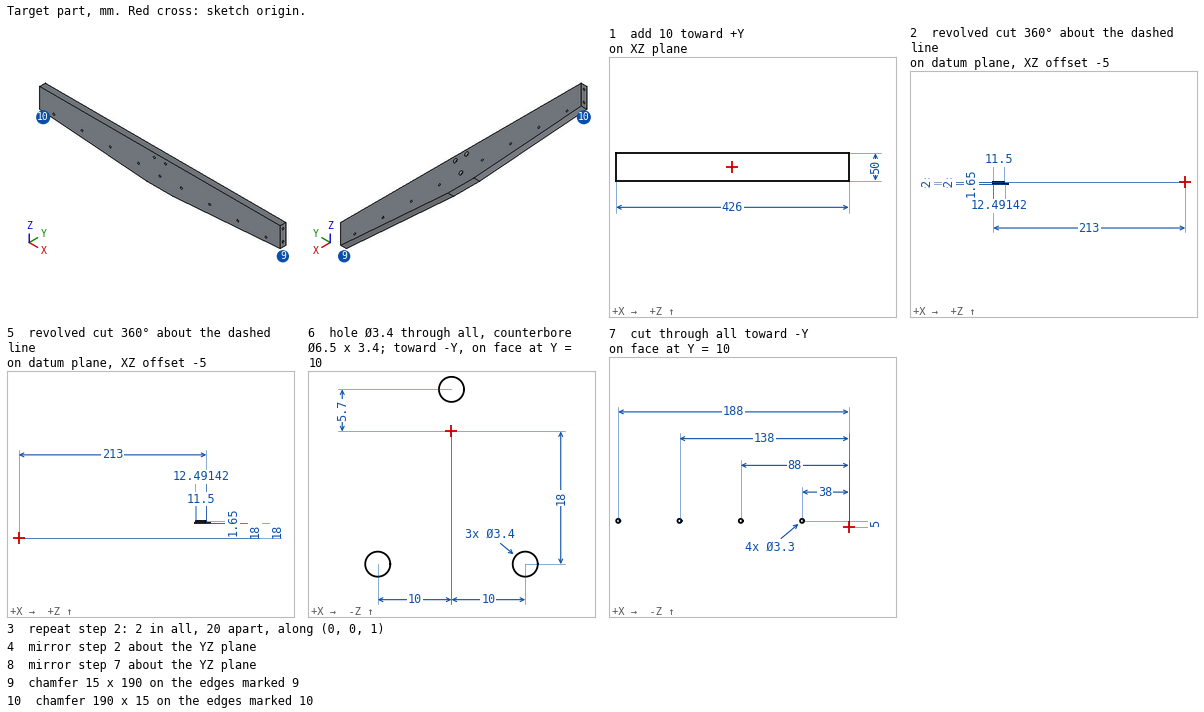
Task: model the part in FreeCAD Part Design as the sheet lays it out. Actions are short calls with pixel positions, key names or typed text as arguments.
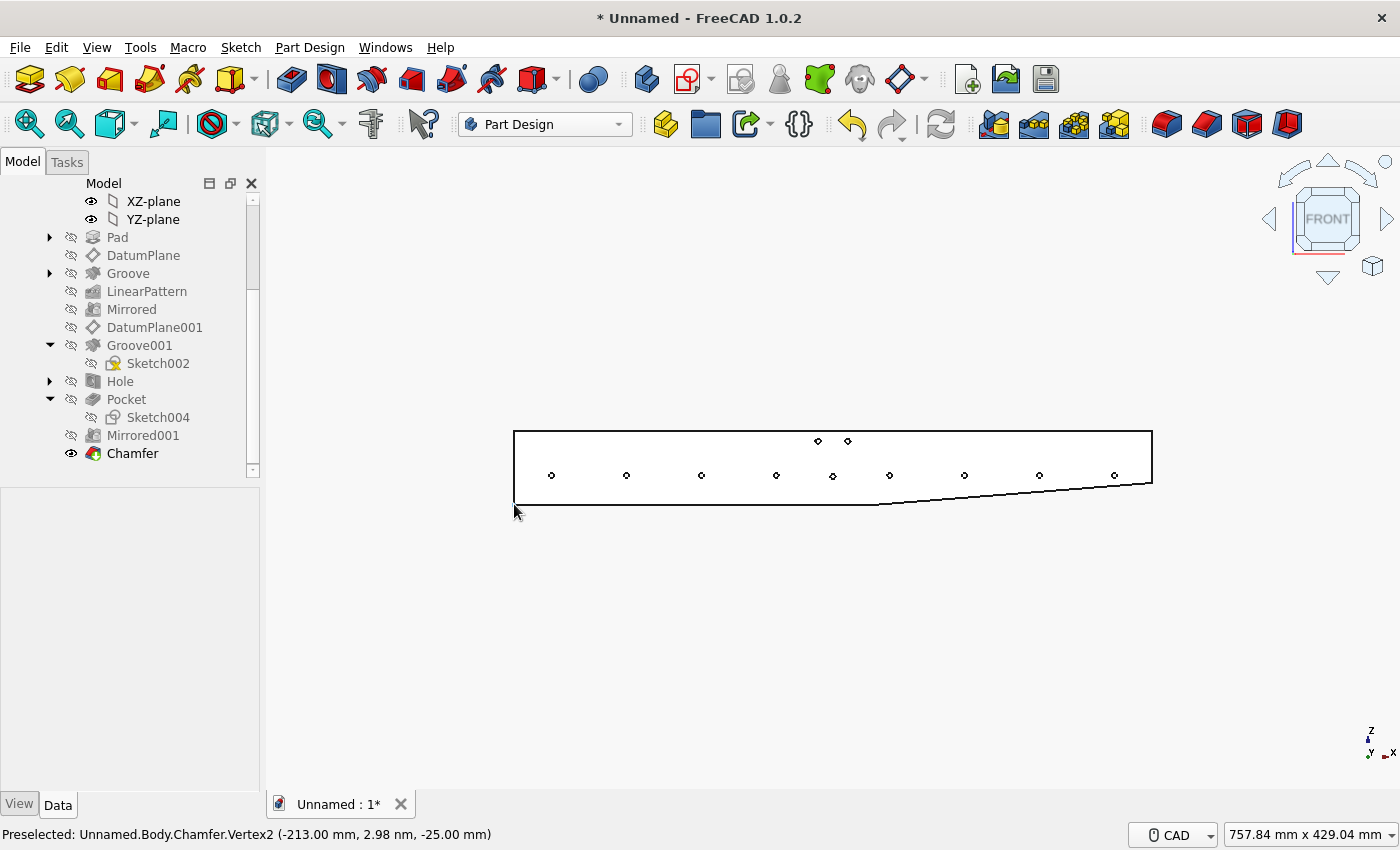
key(3)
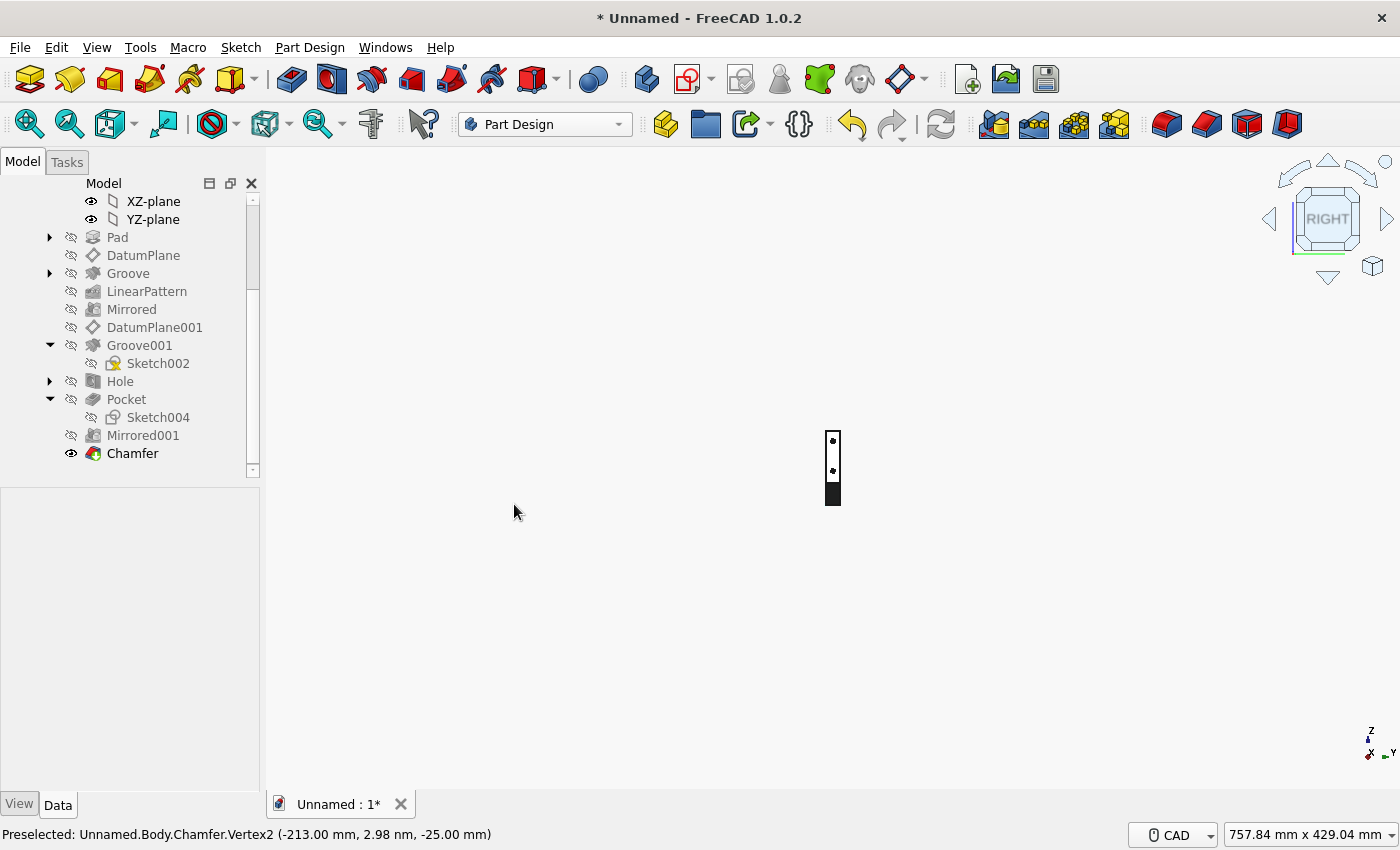
click(30, 124)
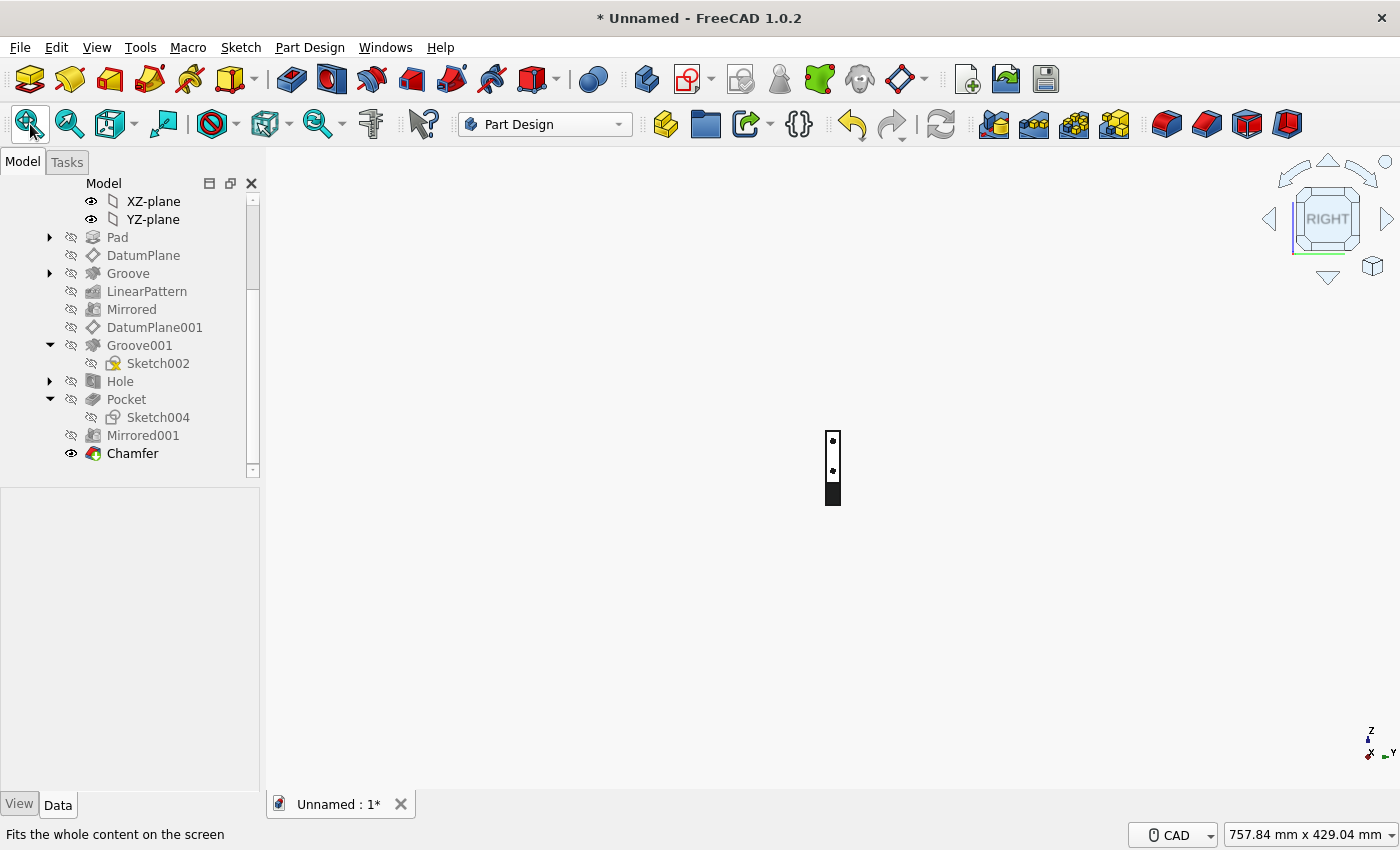
scroll(833, 504, up, 5)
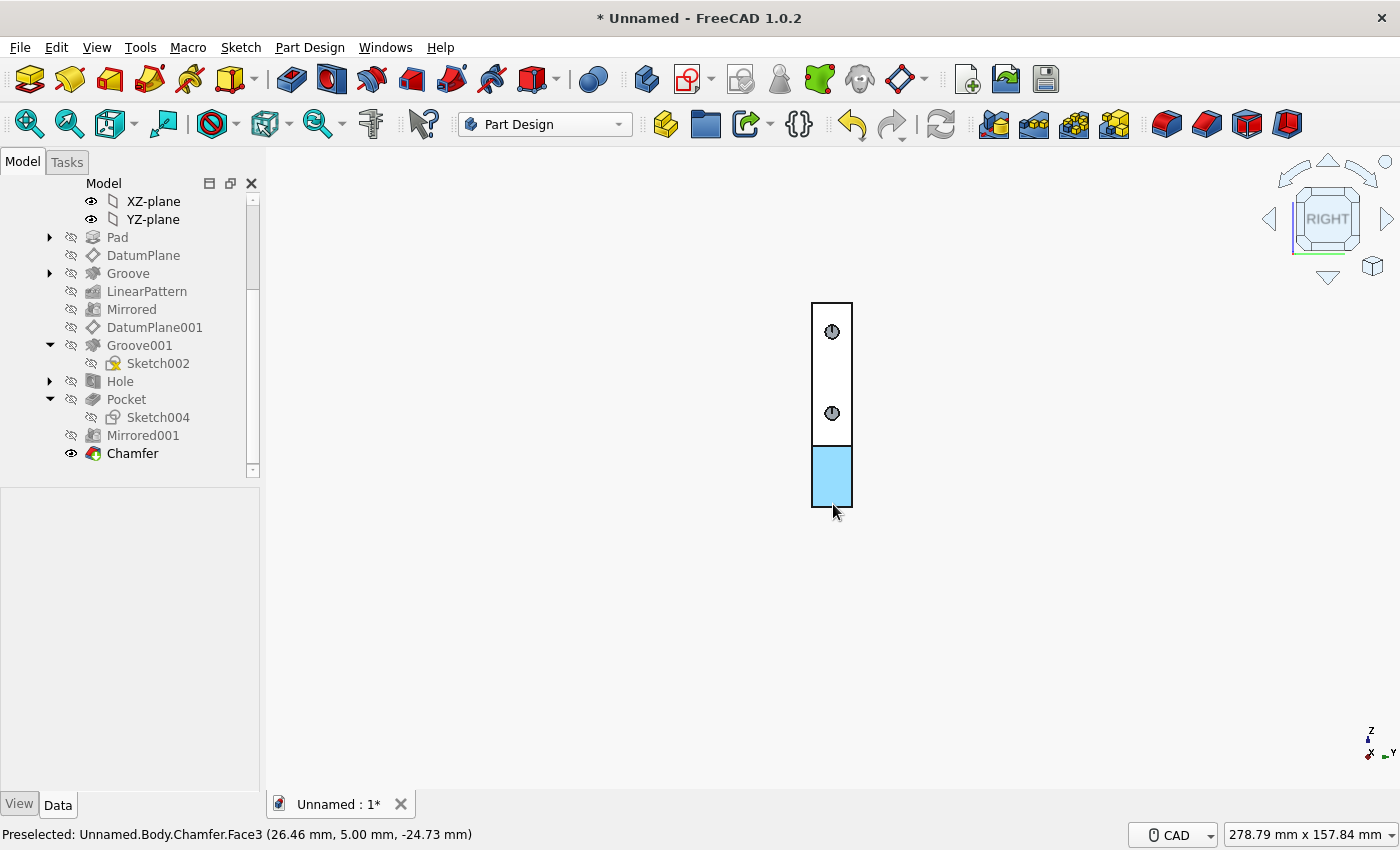
click(30, 124)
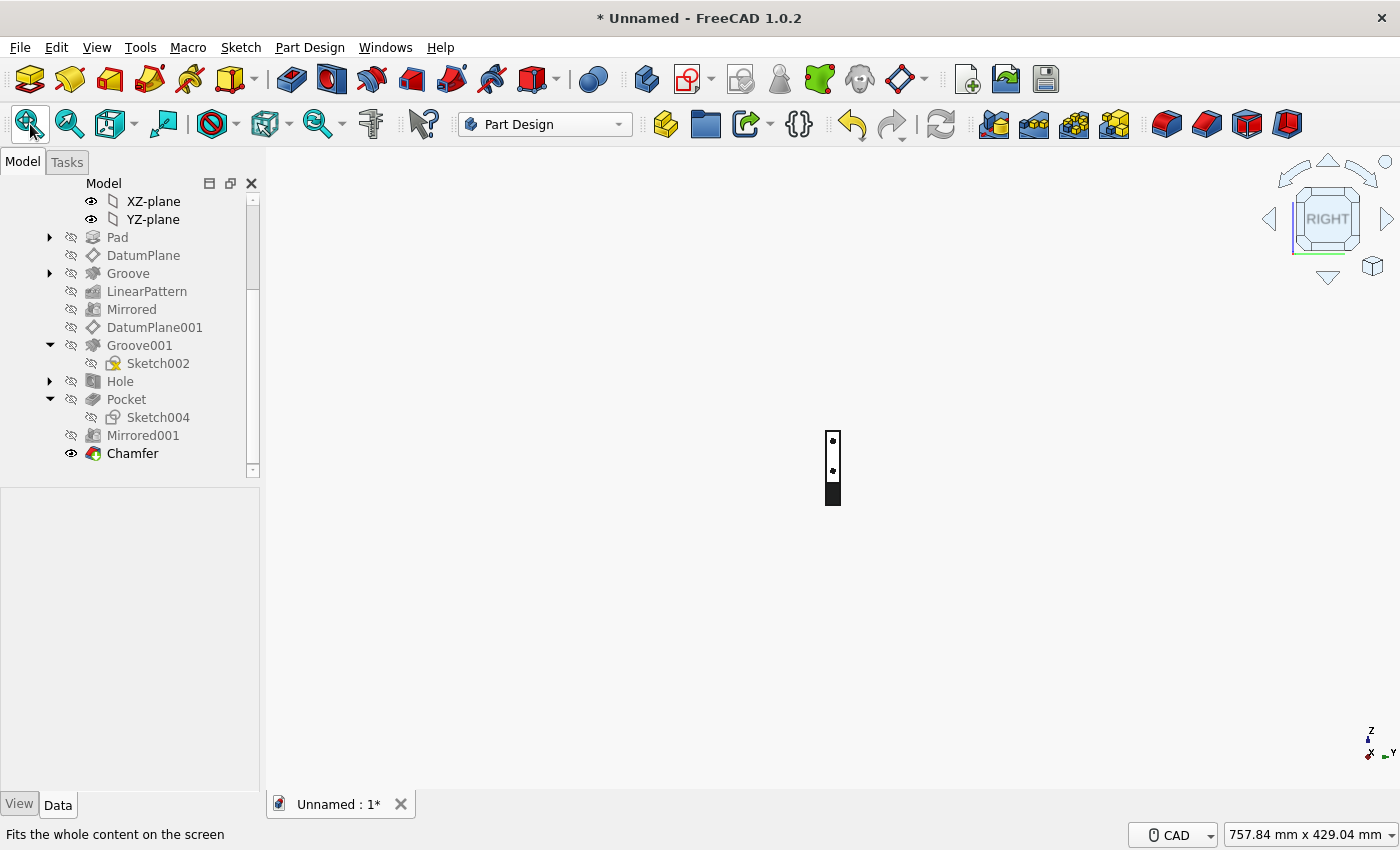
key(5)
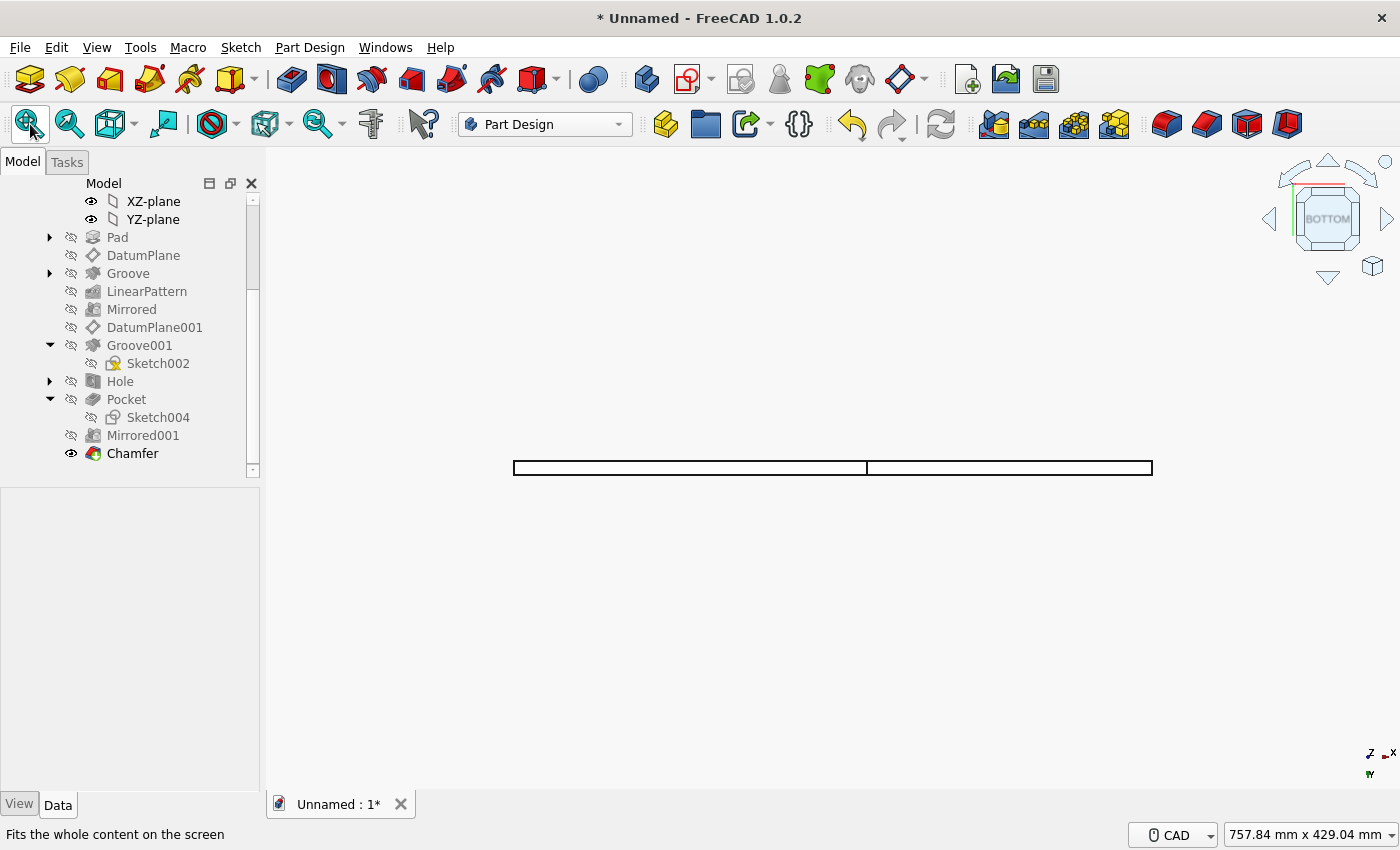
click(514, 467)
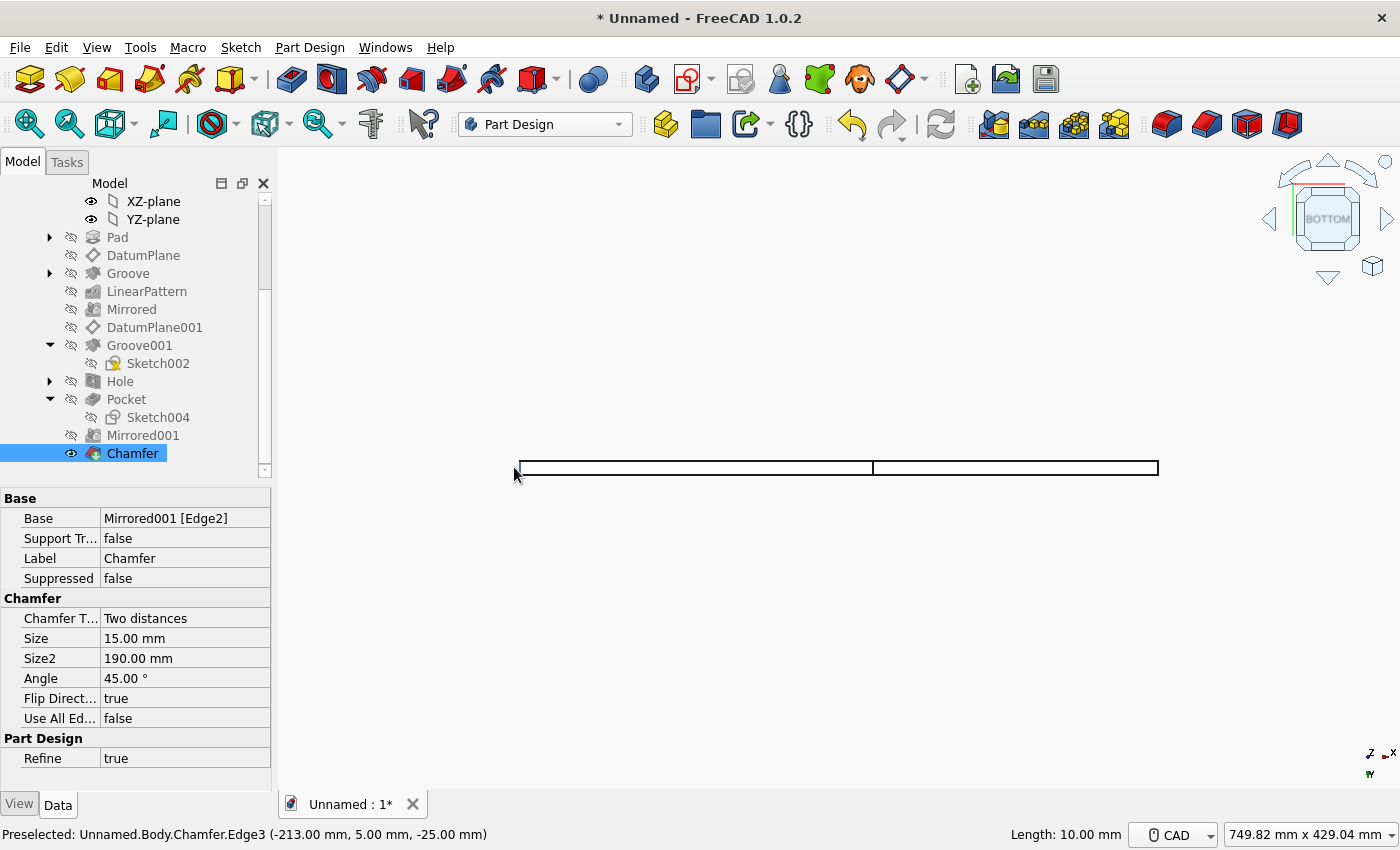
click(1208, 124)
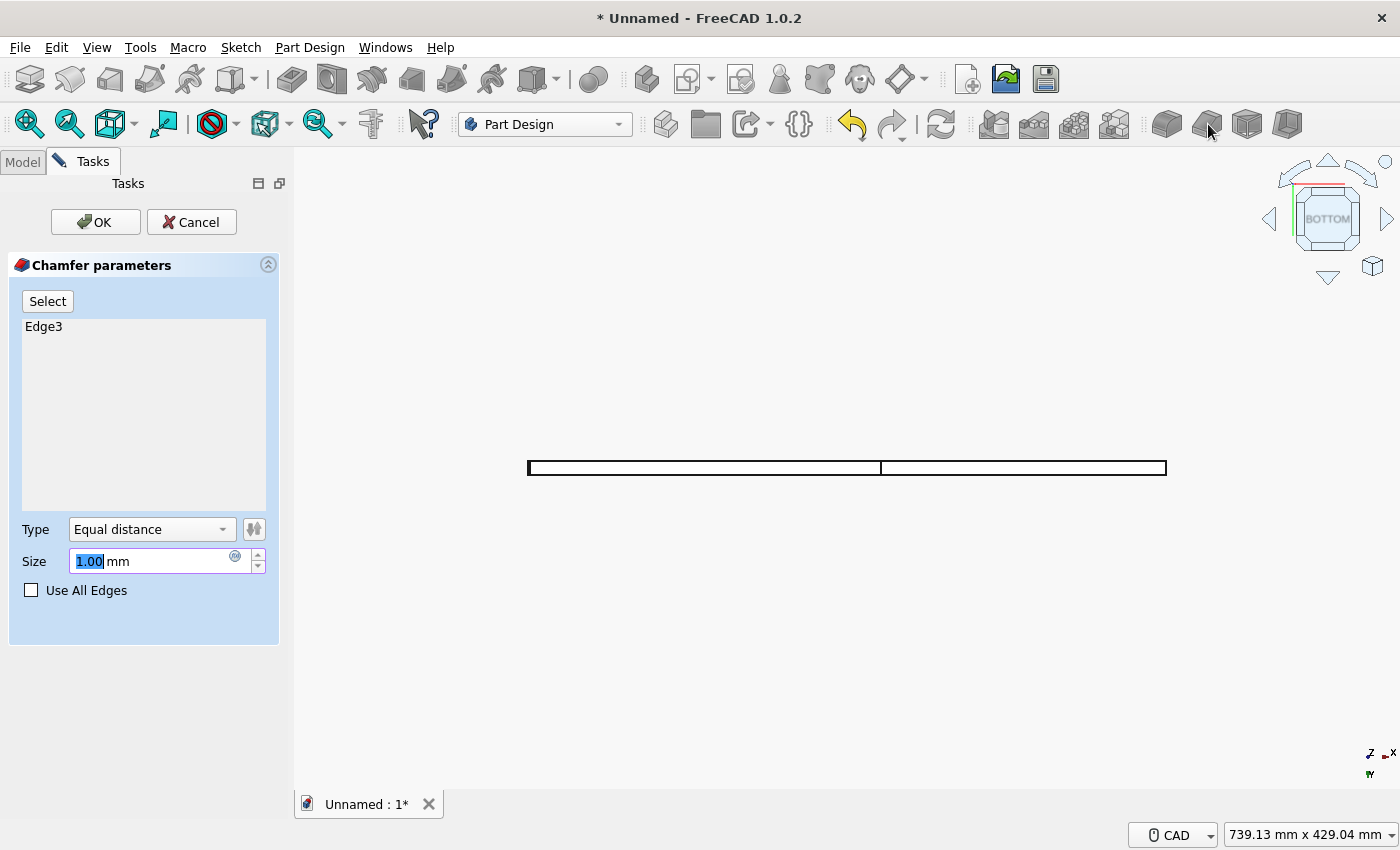
text(190)
key(Tab)